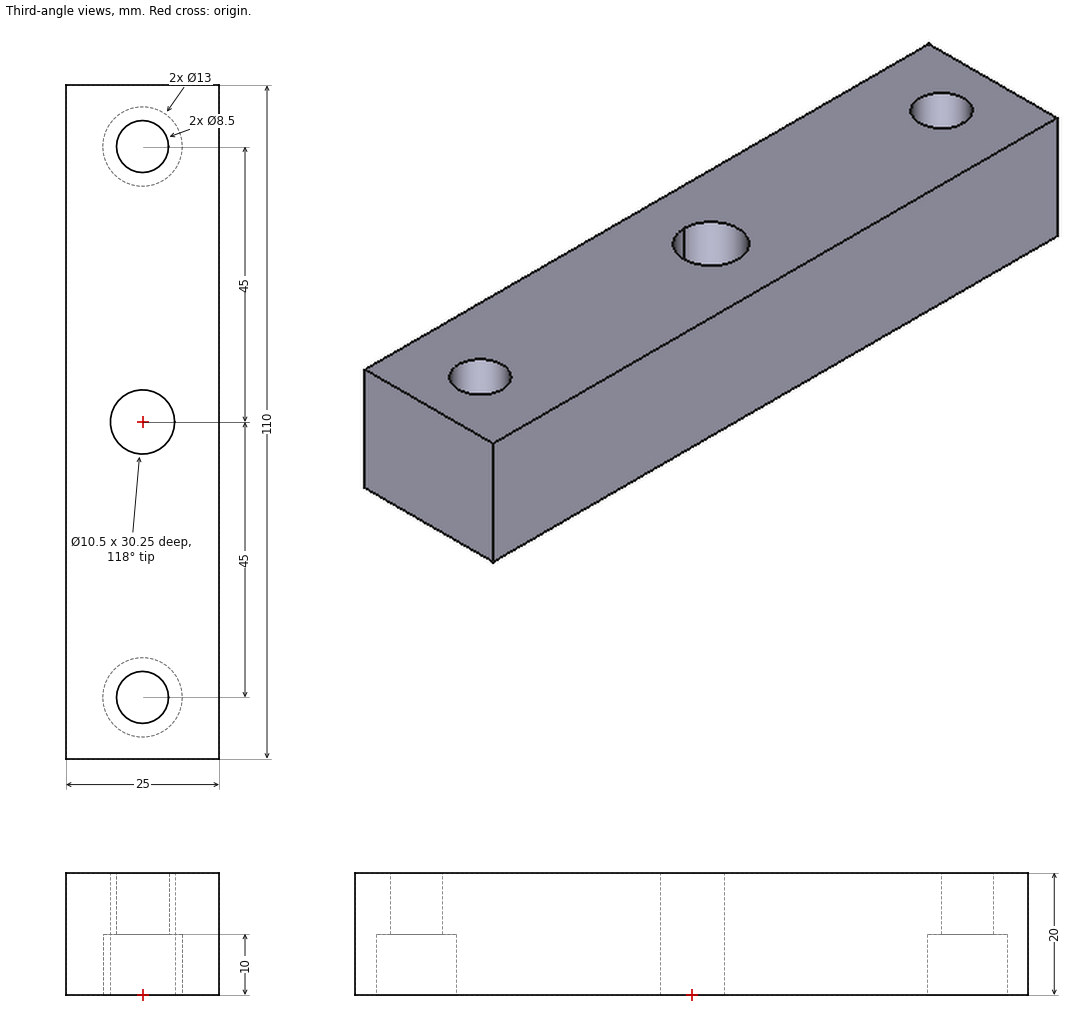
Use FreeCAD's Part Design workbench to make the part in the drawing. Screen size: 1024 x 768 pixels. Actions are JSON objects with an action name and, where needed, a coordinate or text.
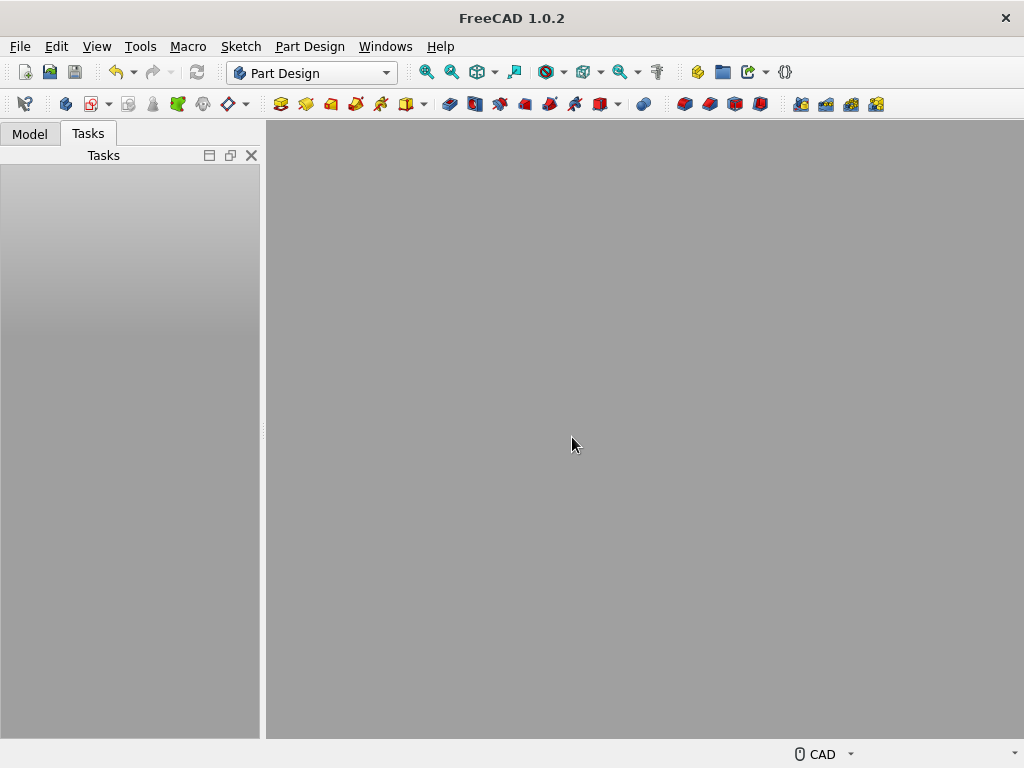
{"action": "left_click", "coordinate": [25, 72]}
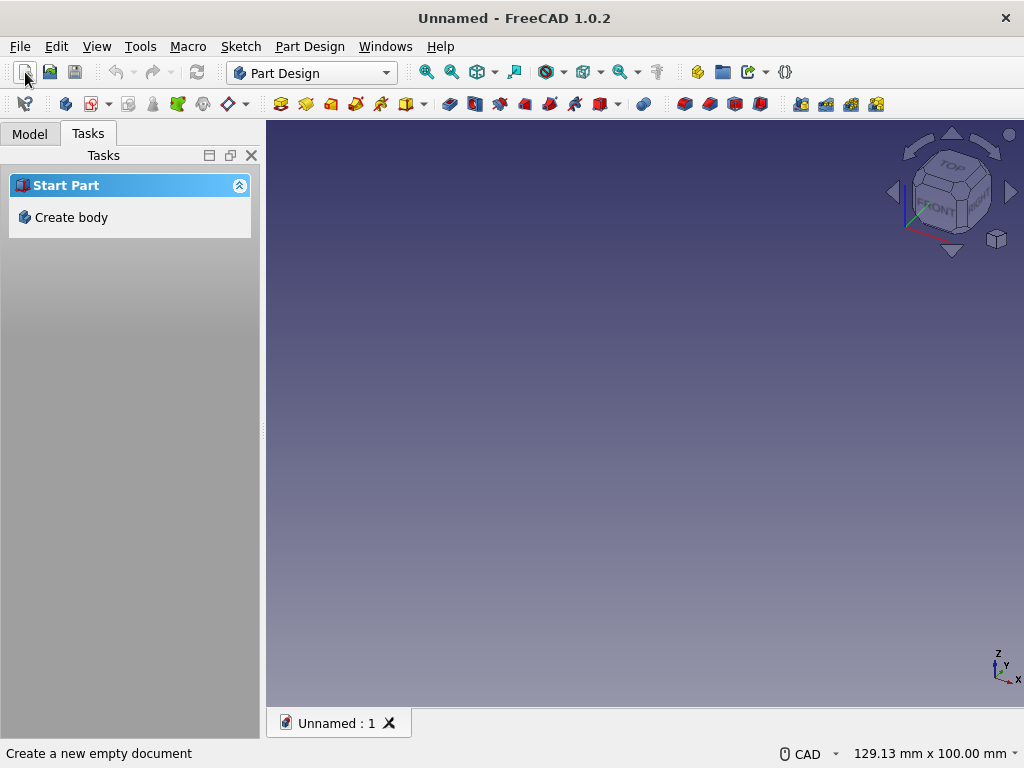
{"action": "left_click", "coordinate": [90, 104]}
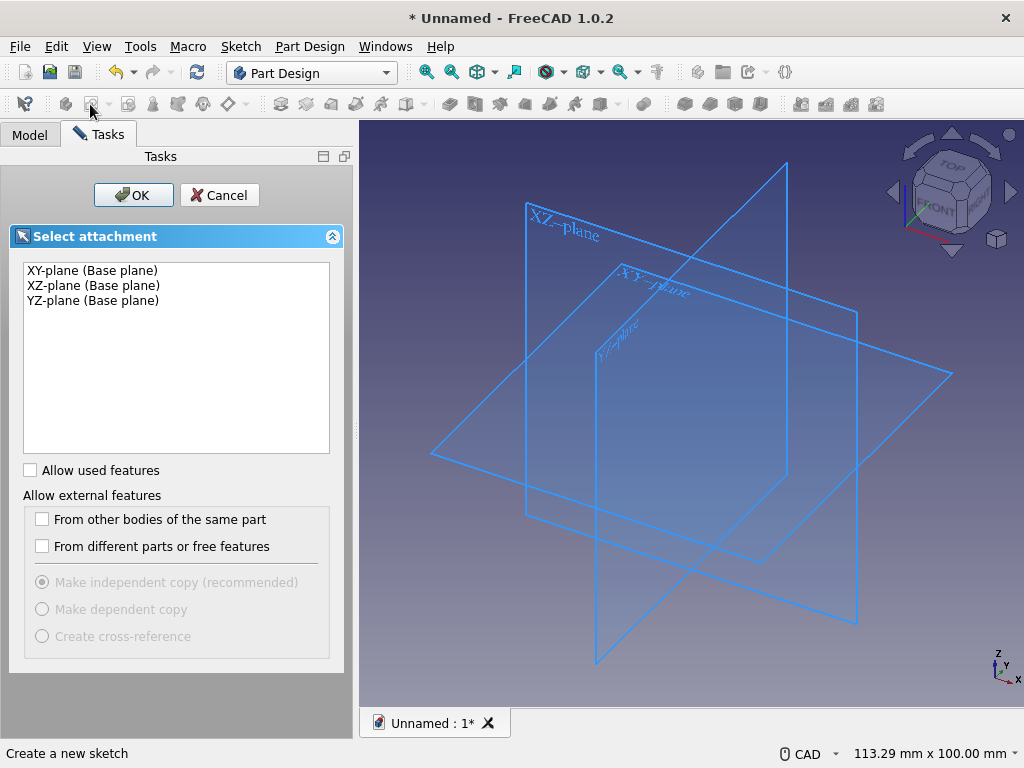
{"action": "left_click", "coordinate": [84, 270]}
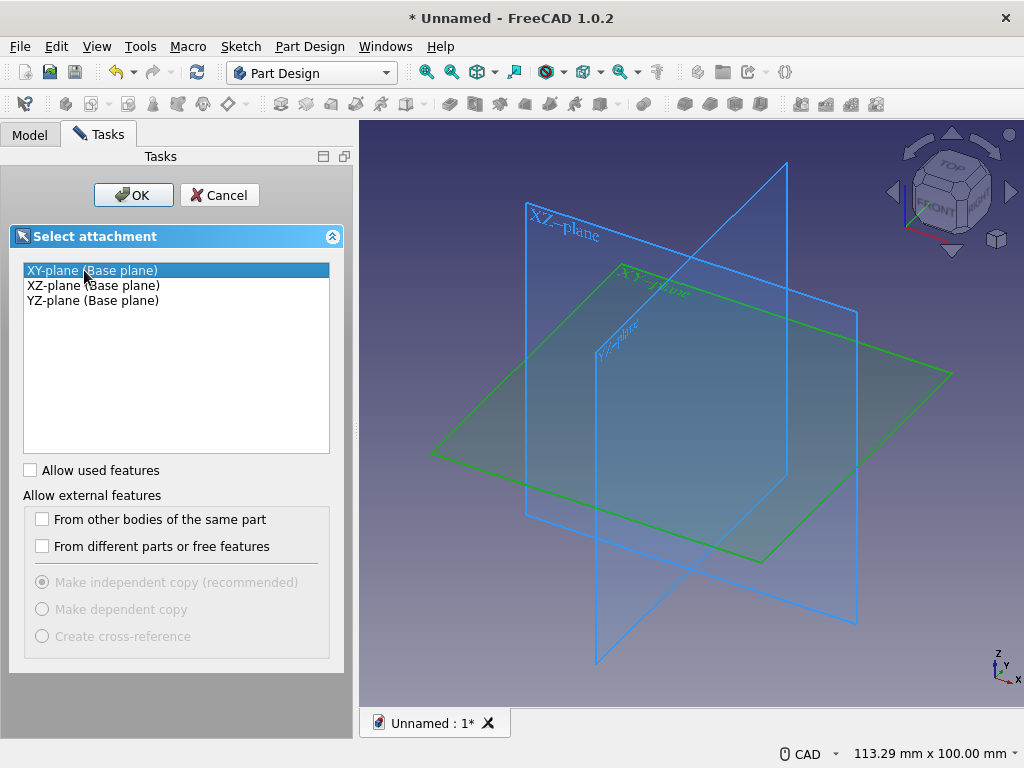
{"action": "left_click", "coordinate": [134, 195]}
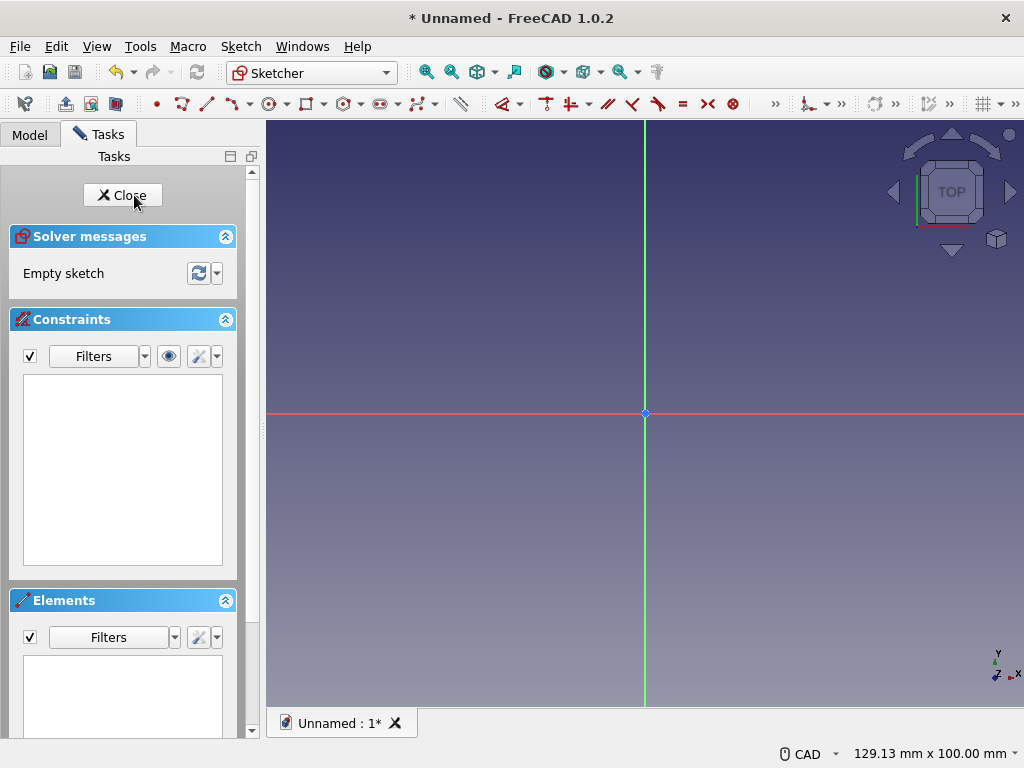
{"action": "scroll", "coordinate": [493, 414], "scroll_direction": "down", "scroll_amount": 3}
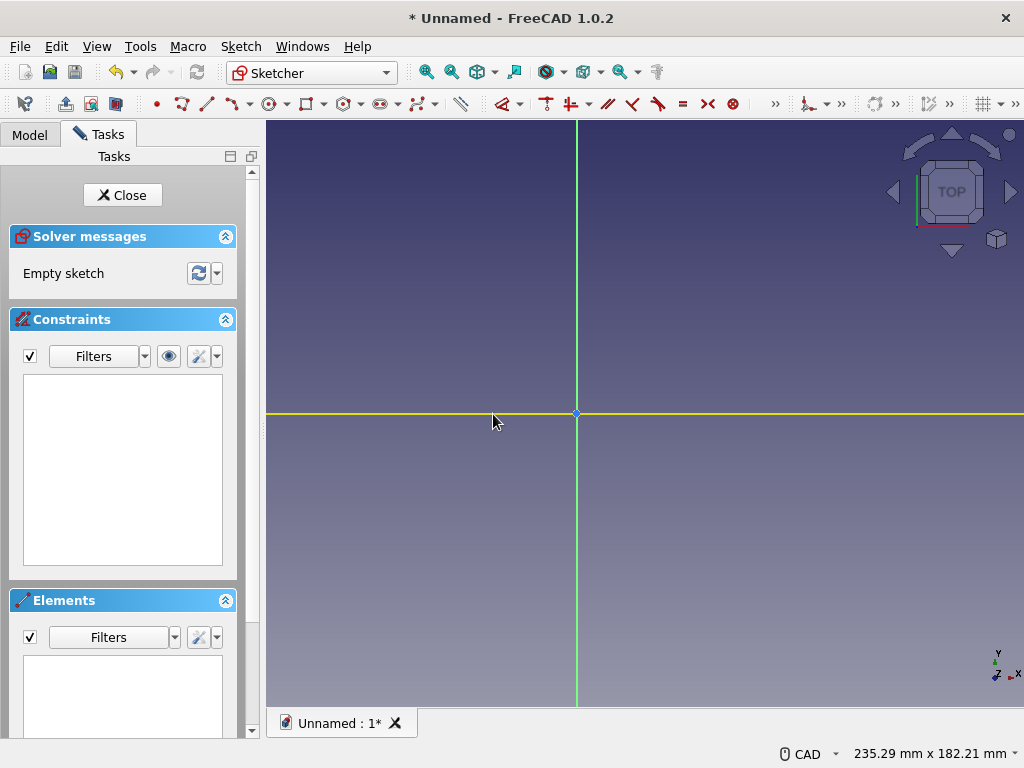
{"action": "key", "text": "g v"}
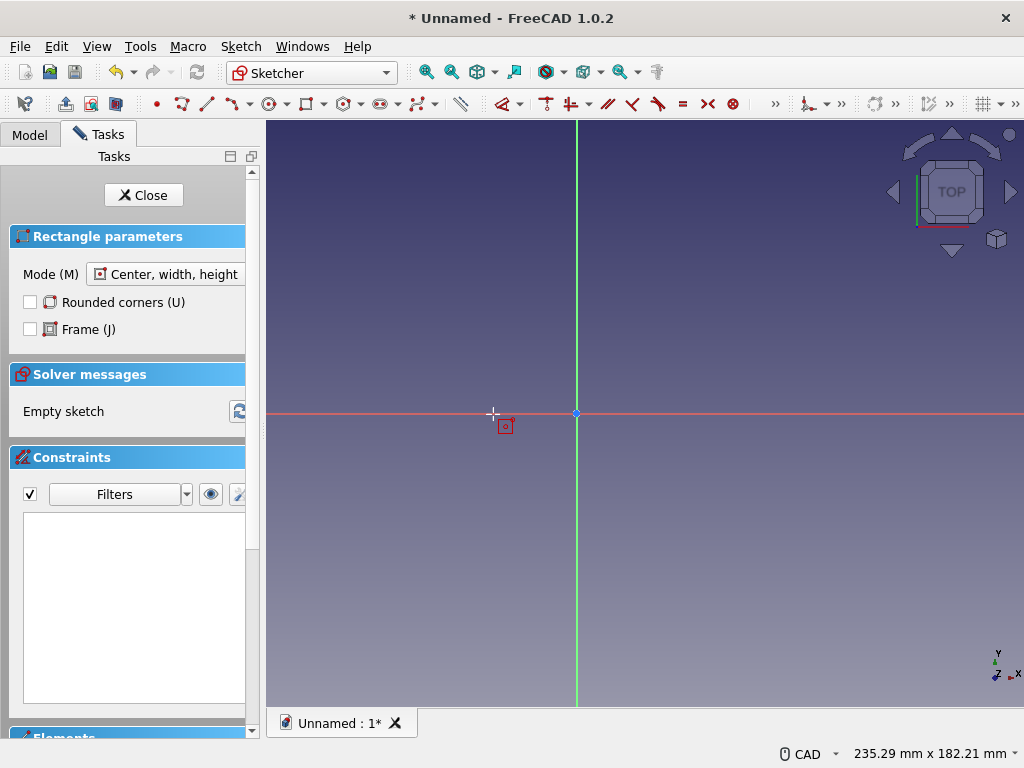
{"action": "left_click", "coordinate": [577, 414]}
{"action": "left_click", "coordinate": [617, 237]}
{"action": "key", "text": "Escape"}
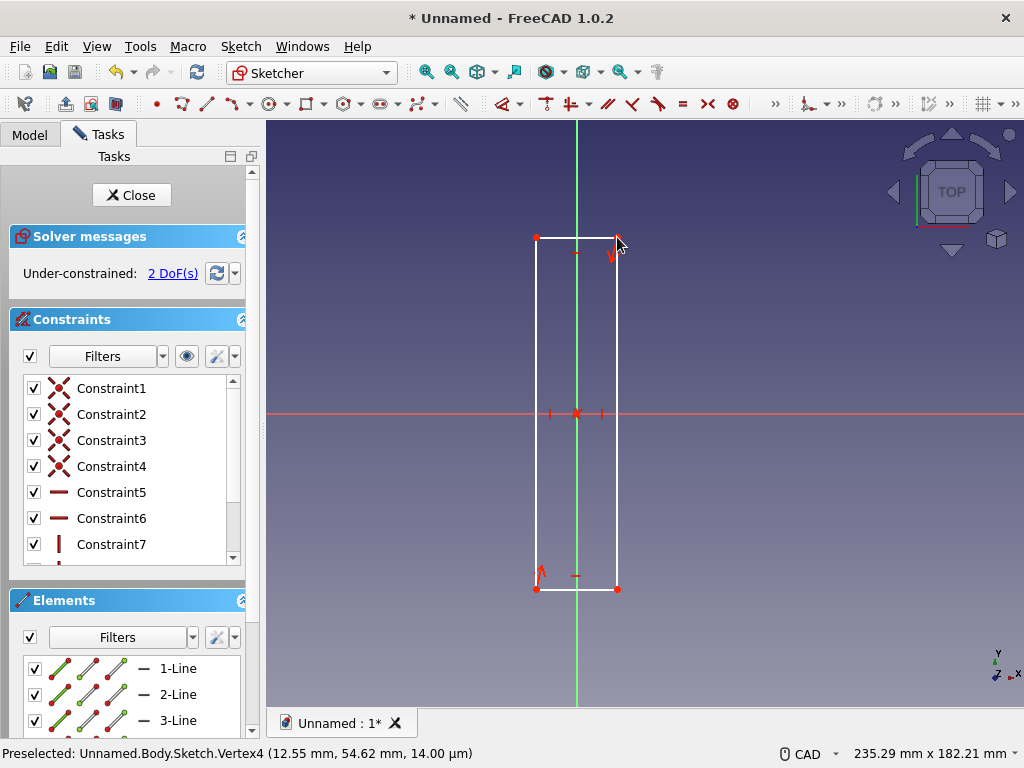
{"action": "key", "text": "d"}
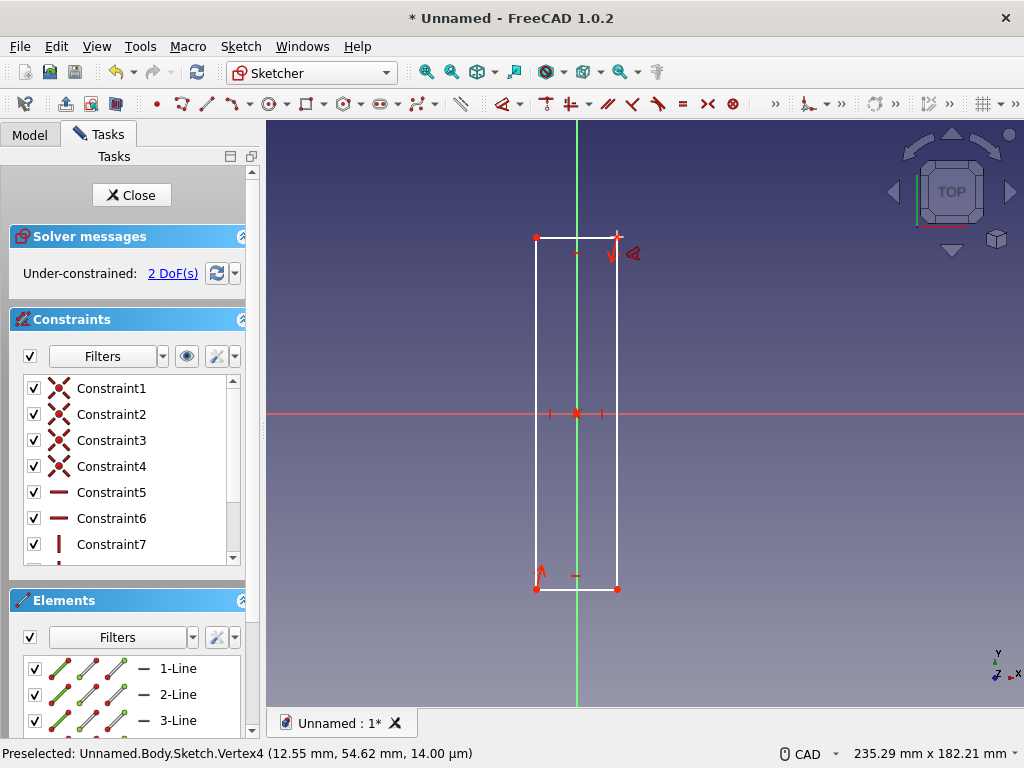
{"action": "left_click", "coordinate": [560, 590]}
{"action": "left_click", "coordinate": [558, 624]}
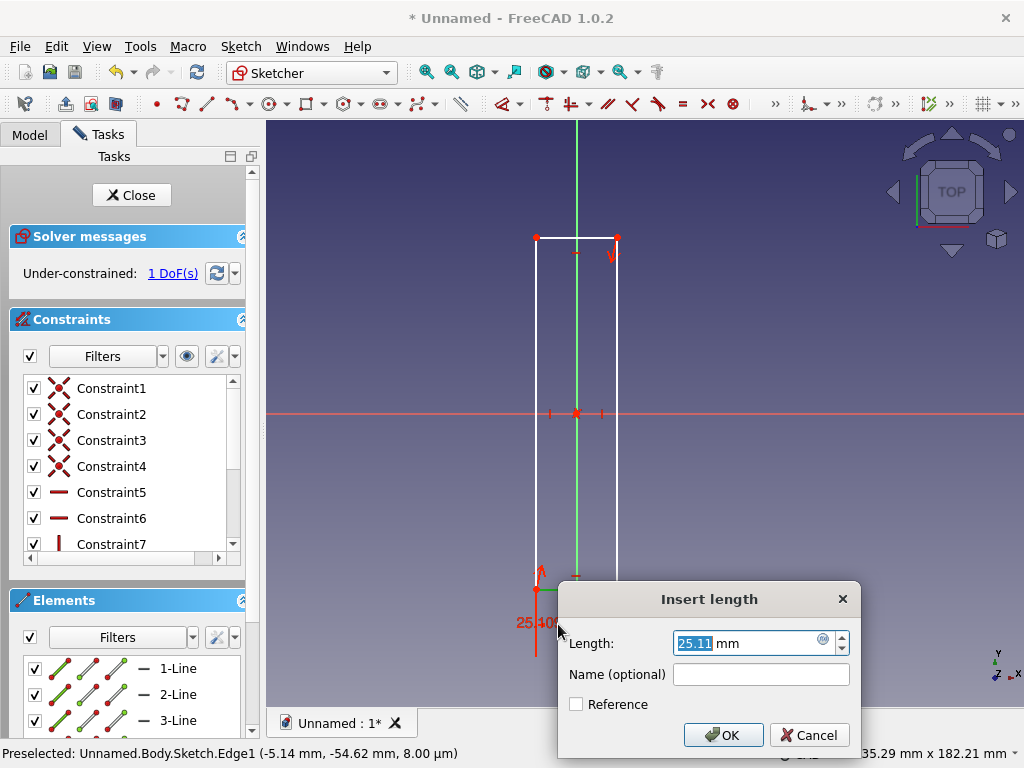
{"action": "type", "text": "25"}
{"action": "key", "text": "Return"}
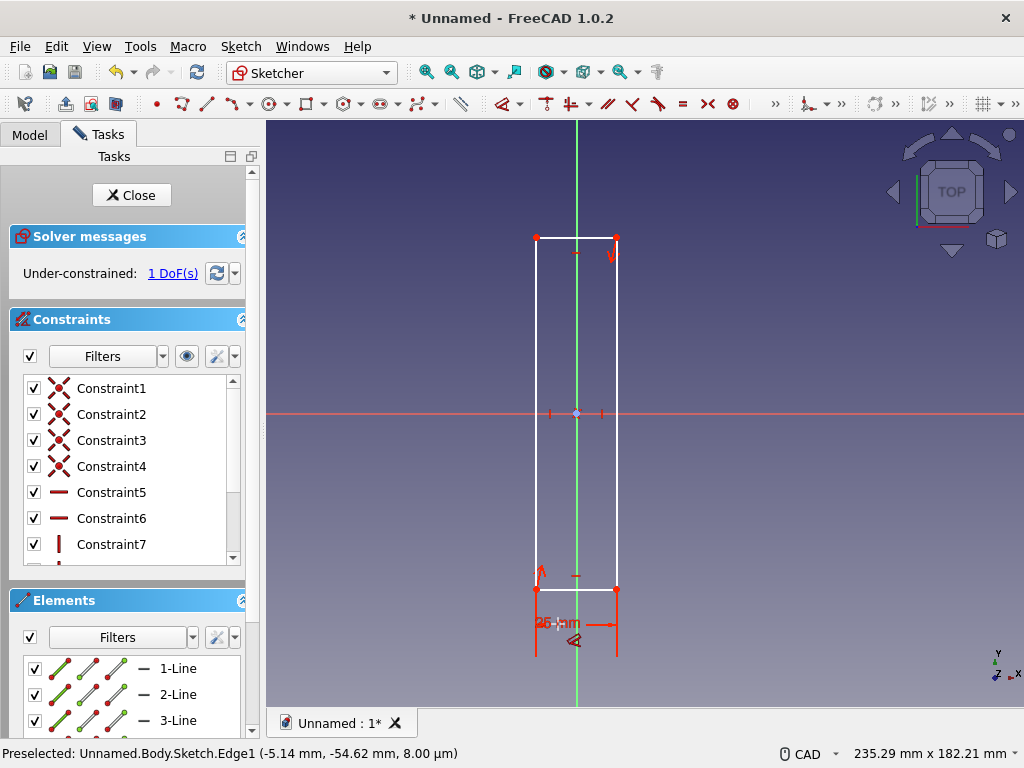
{"action": "left_click", "coordinate": [617, 484]}
{"action": "left_click", "coordinate": [651, 333]}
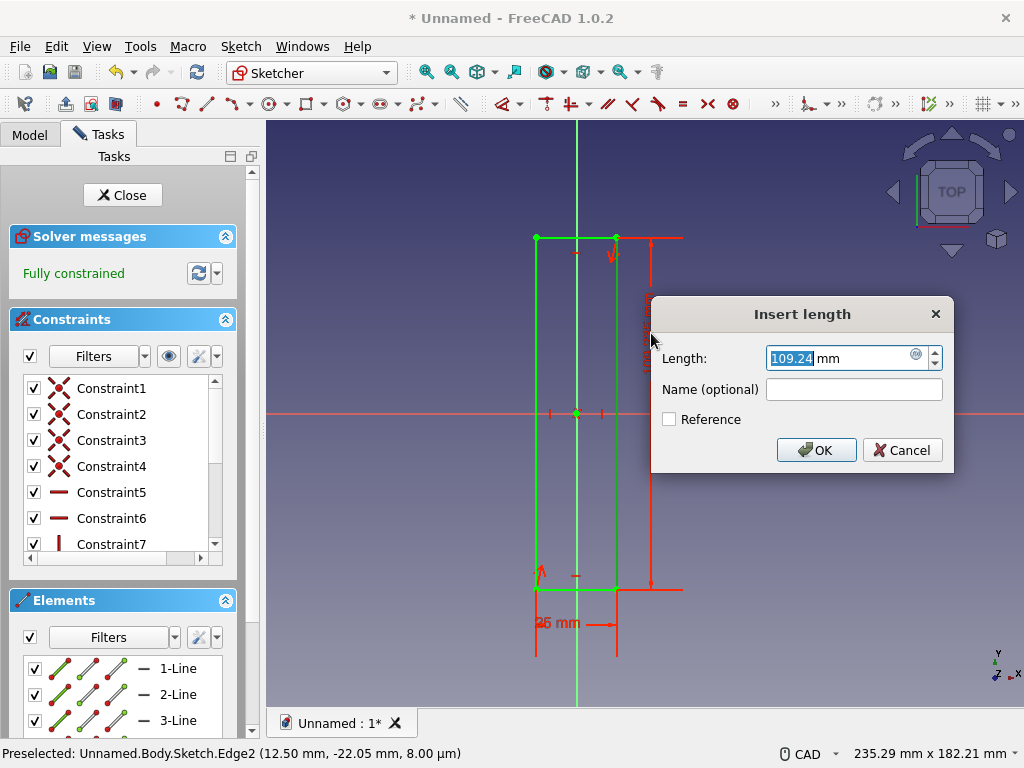
{"action": "type", "text": "110"}
{"action": "key", "text": "Return"}
{"action": "key", "text": "Escape"}